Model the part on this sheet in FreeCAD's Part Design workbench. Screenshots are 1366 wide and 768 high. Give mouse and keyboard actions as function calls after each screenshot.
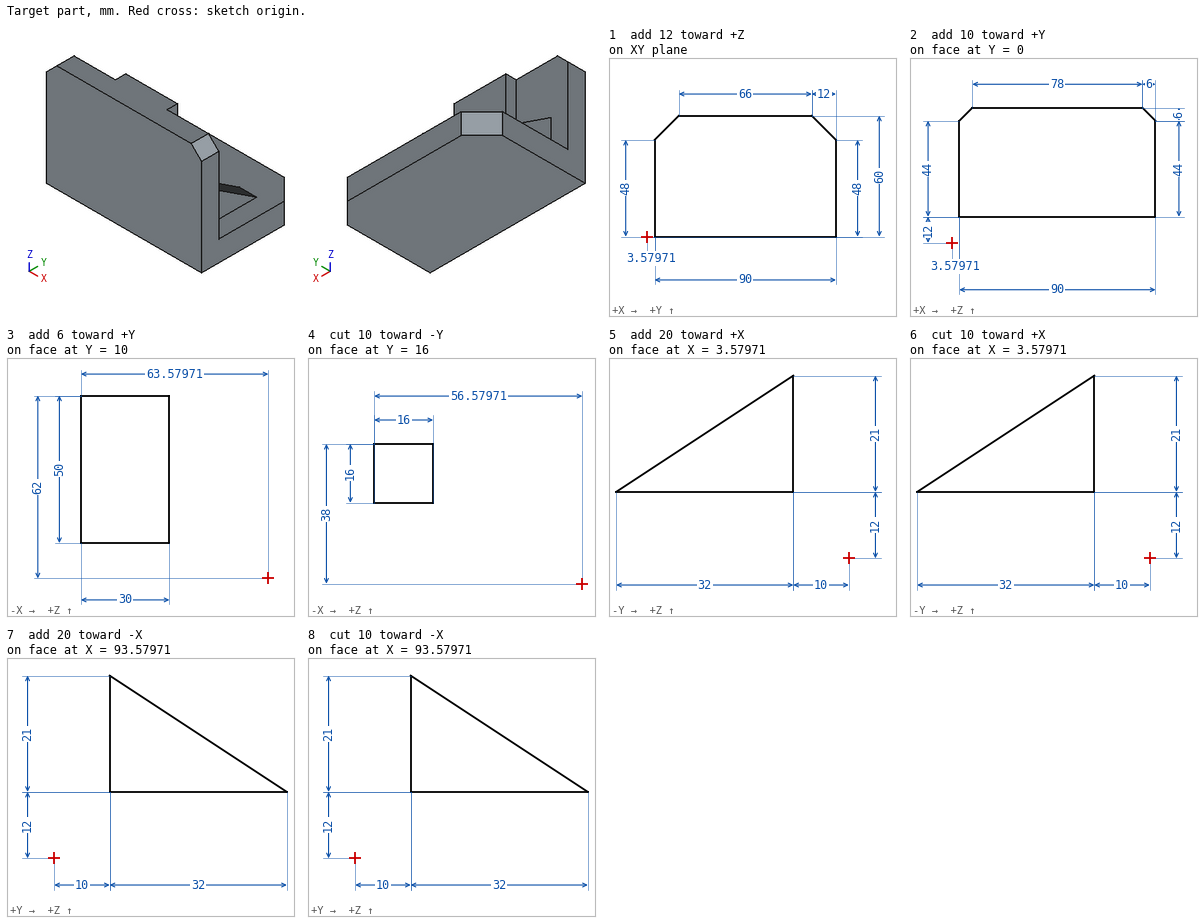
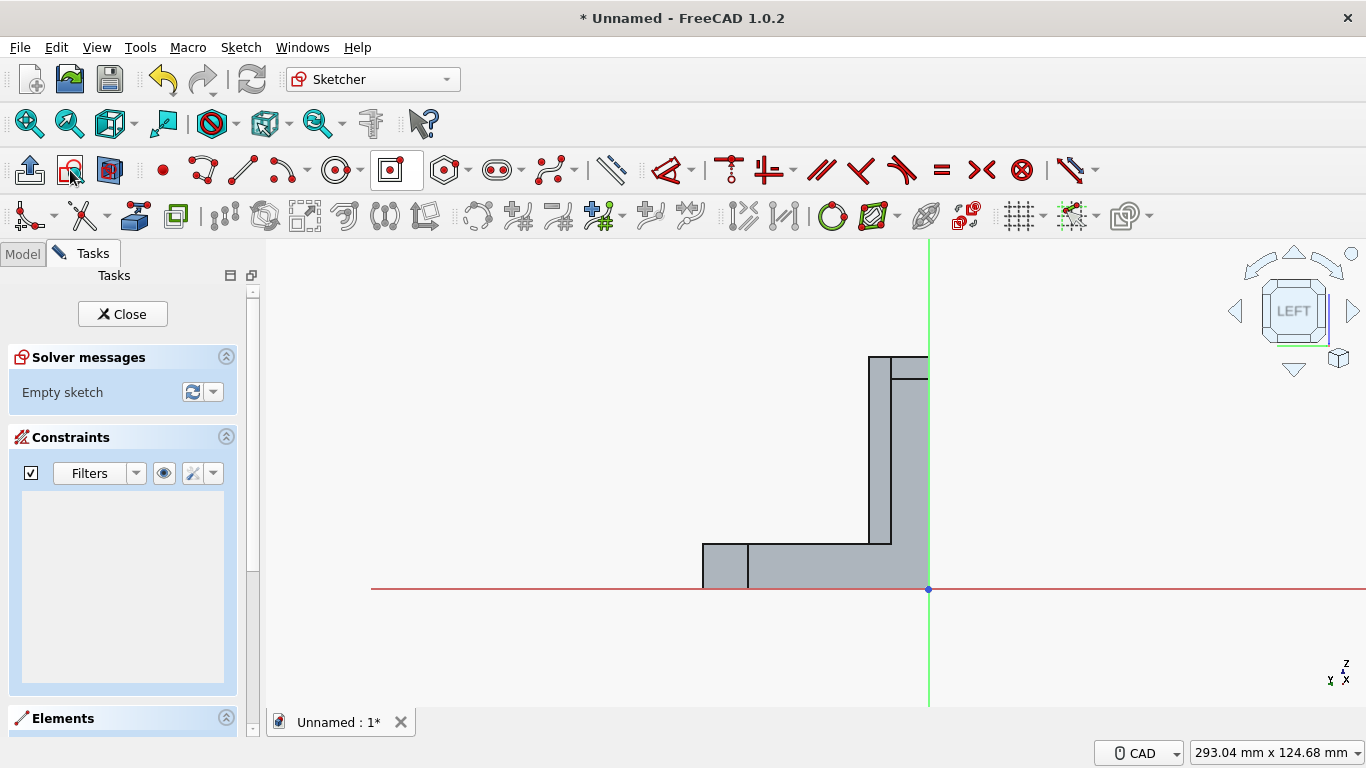
scroll(933, 572, up, 4)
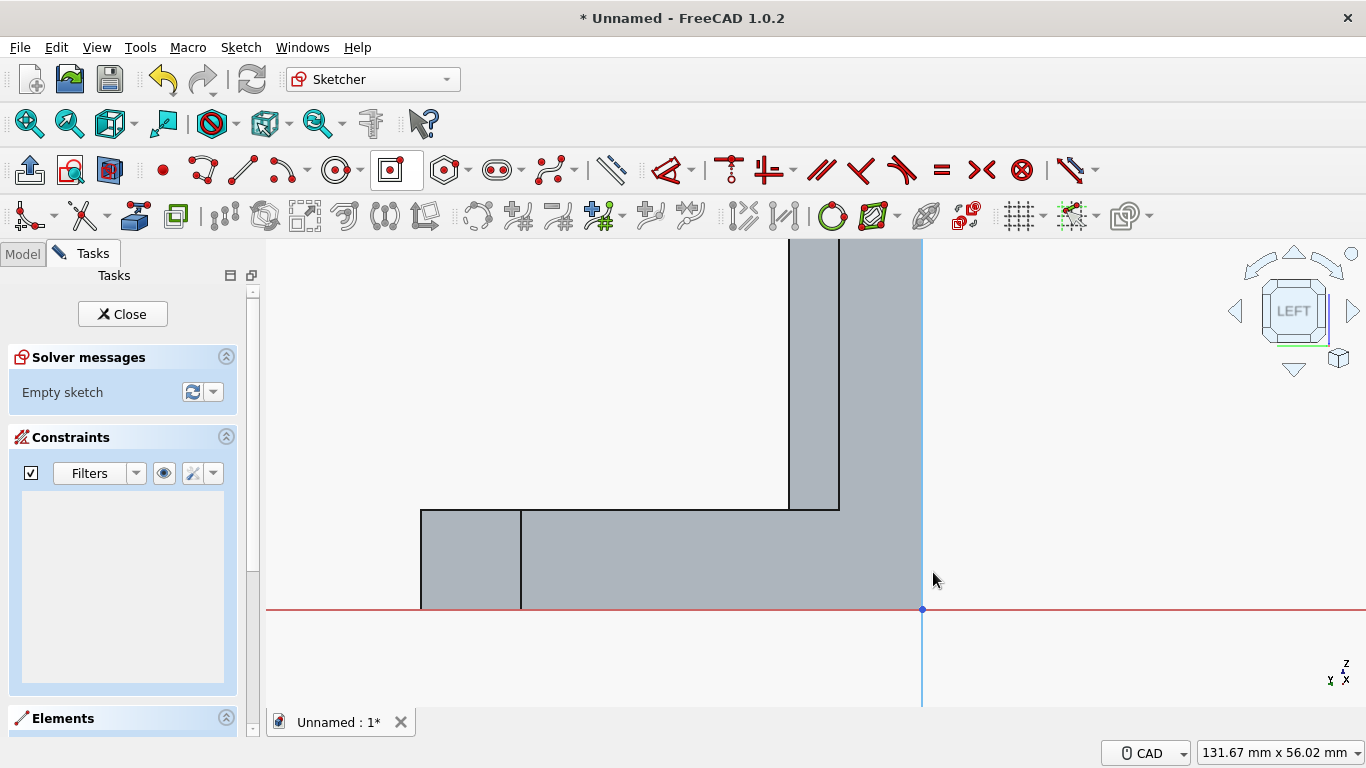
key(g)
key(m)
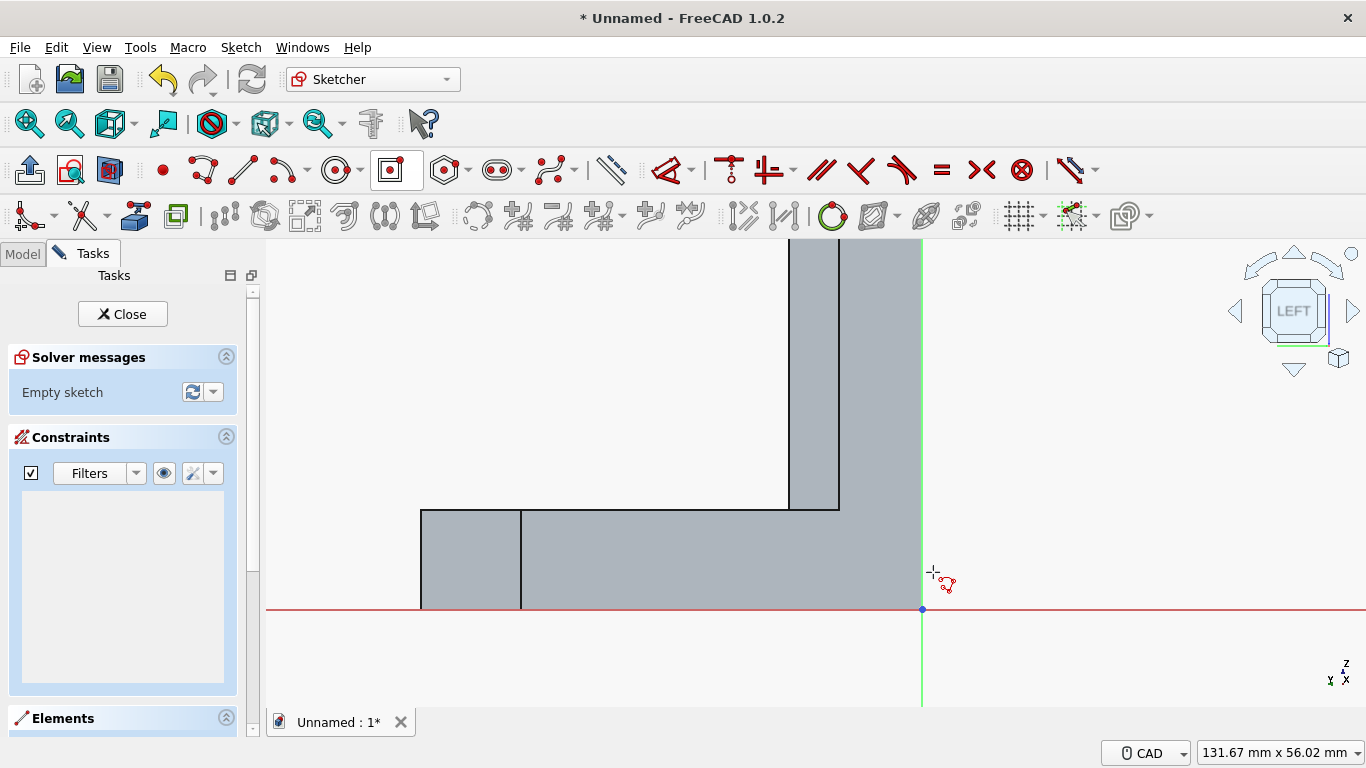
click(839, 510)
click(839, 334)
click(572, 510)
click(839, 511)
key(Escape)
key(Escape)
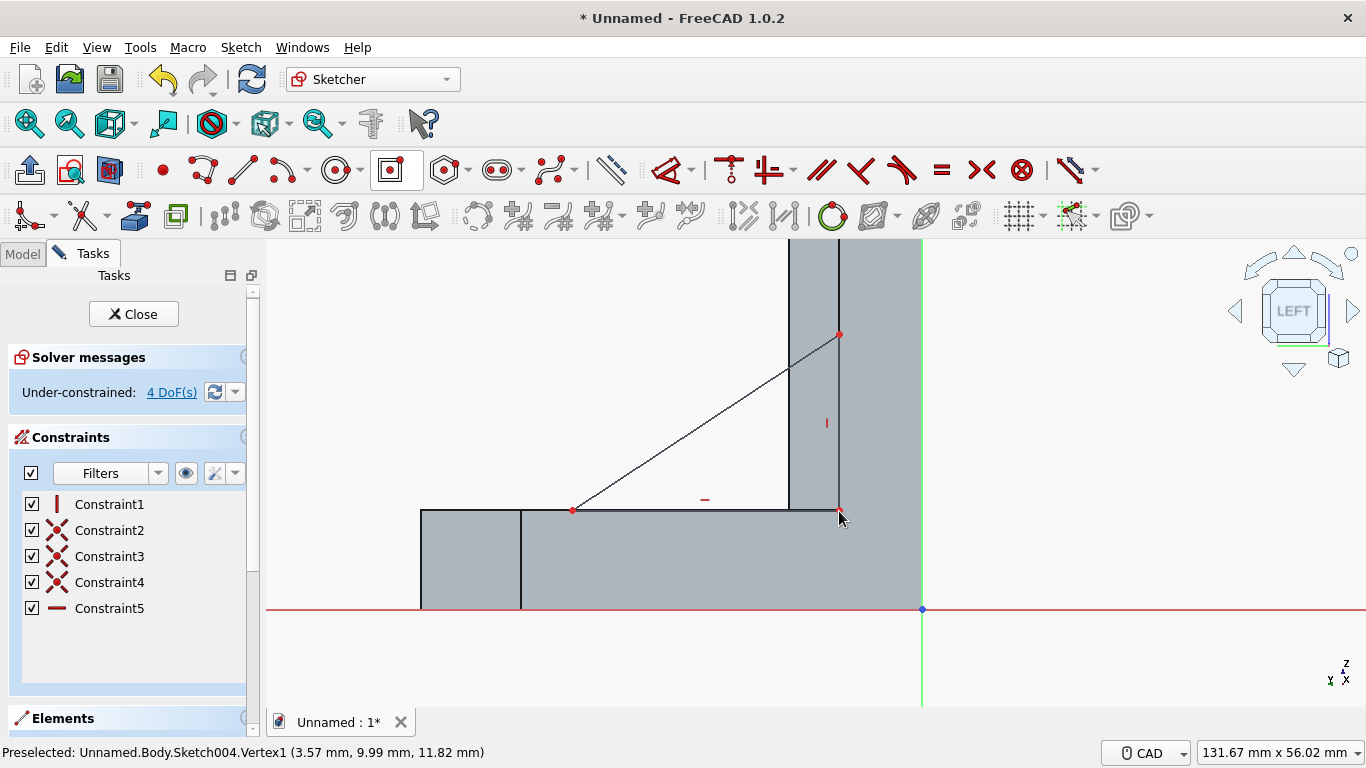
key(d)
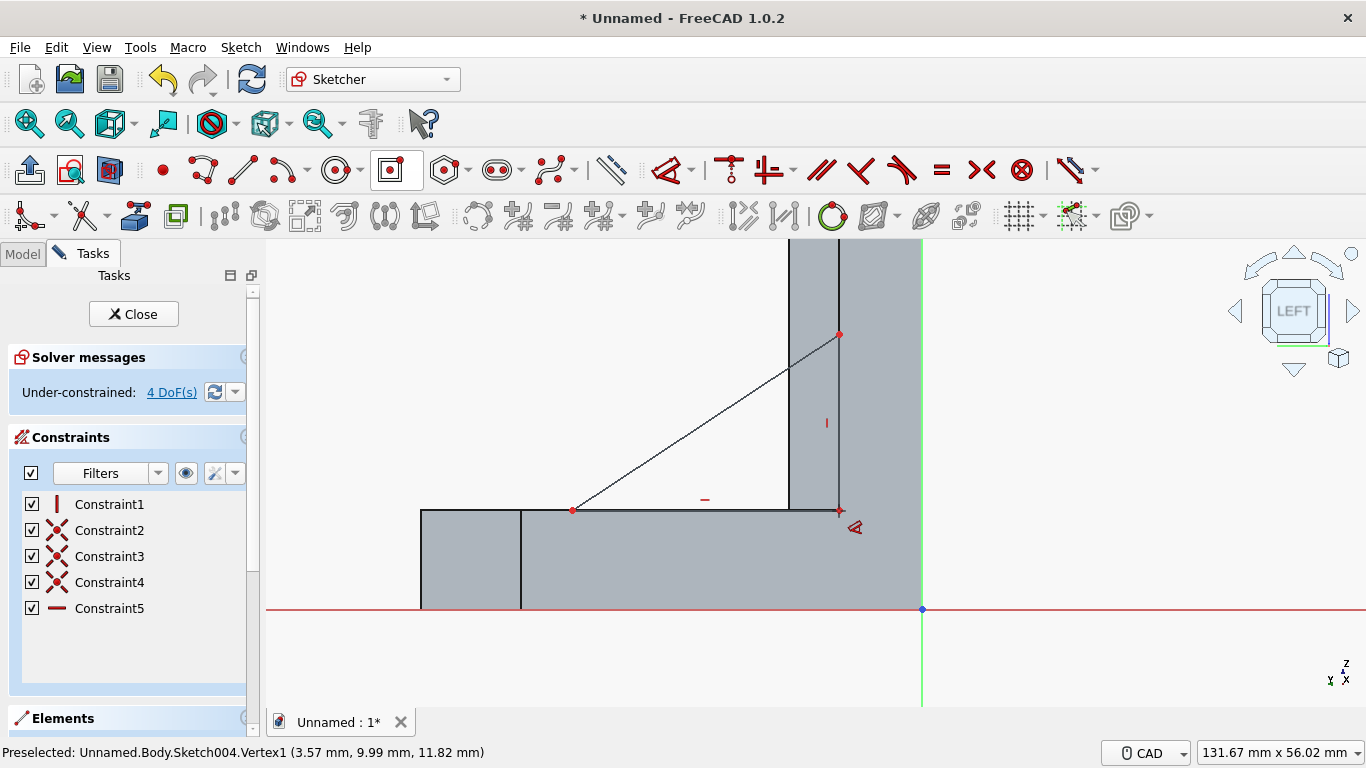
click(839, 458)
click(873, 423)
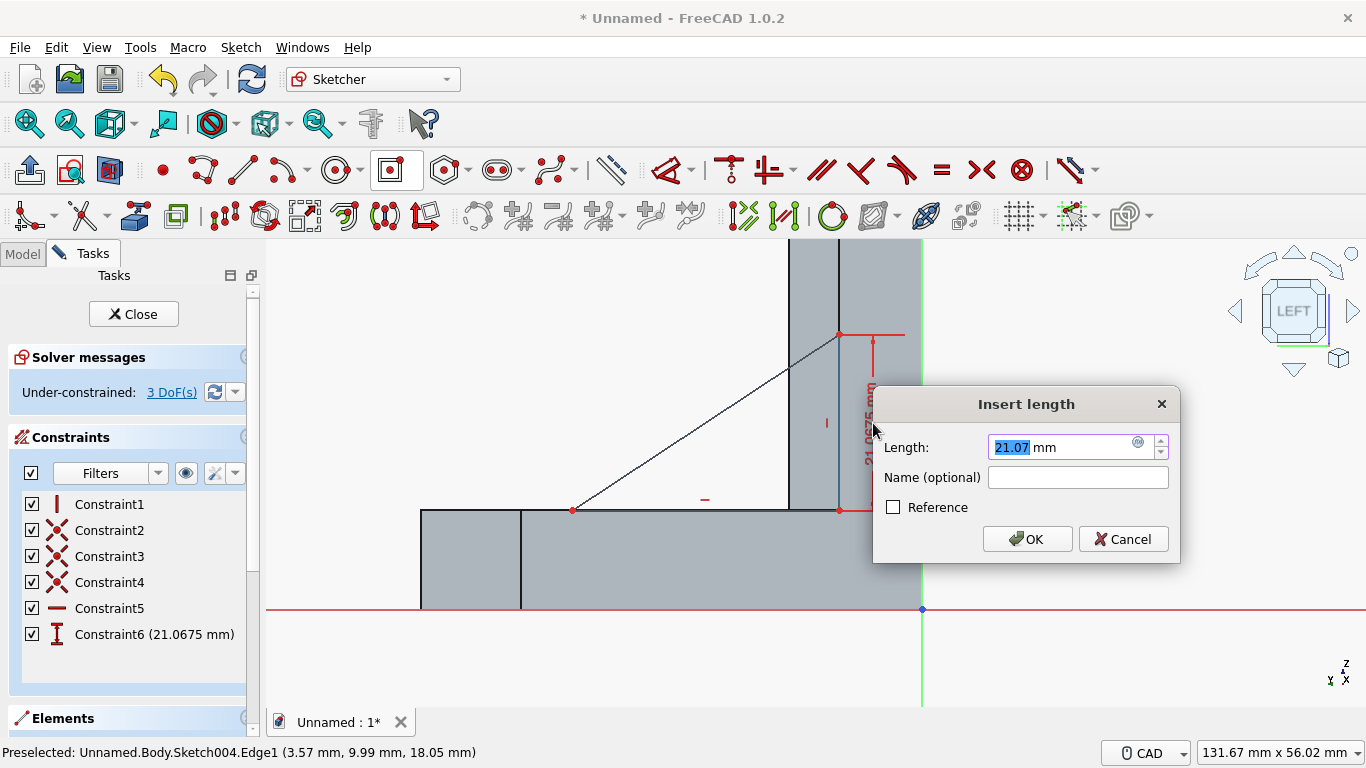
text(21)
key(Return)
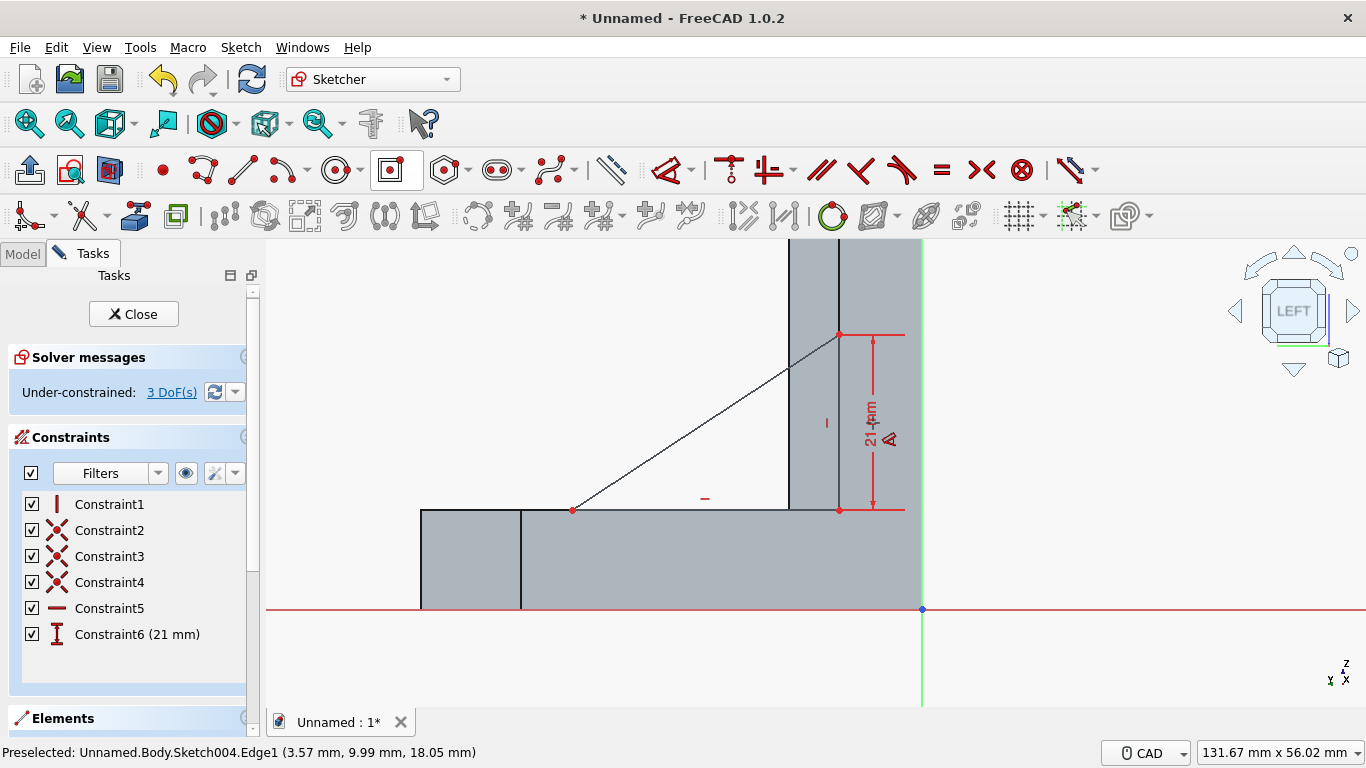
click(652, 510)
click(705, 544)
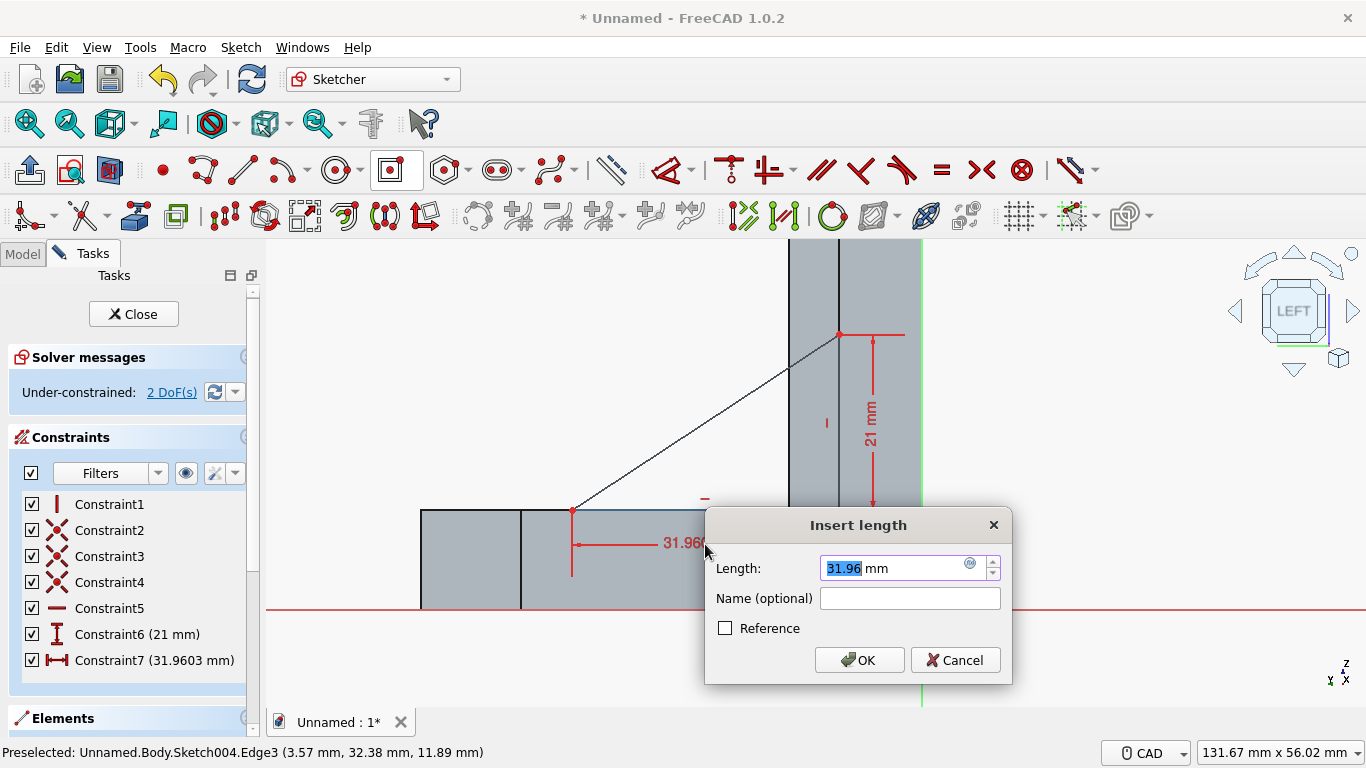
text(32)
key(Return)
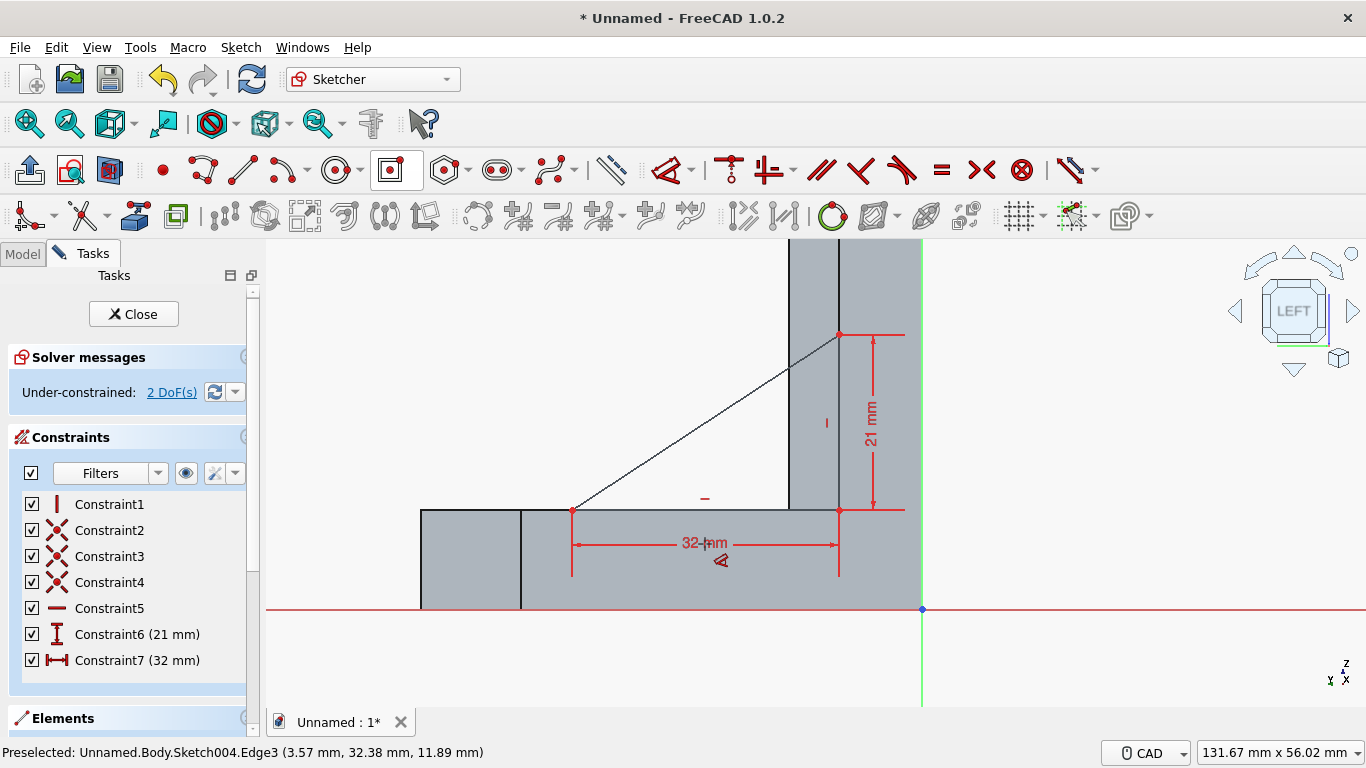
click(839, 510)
click(881, 644)